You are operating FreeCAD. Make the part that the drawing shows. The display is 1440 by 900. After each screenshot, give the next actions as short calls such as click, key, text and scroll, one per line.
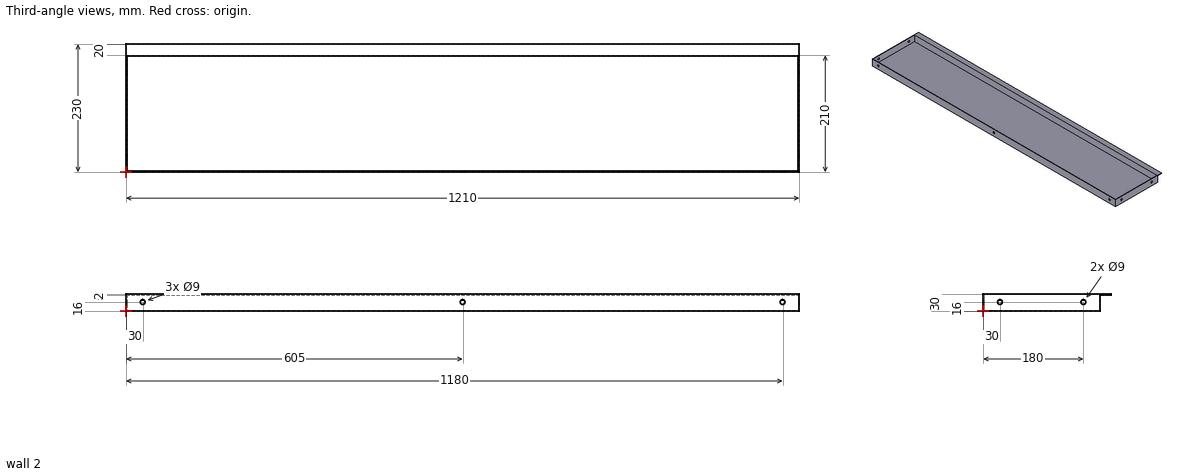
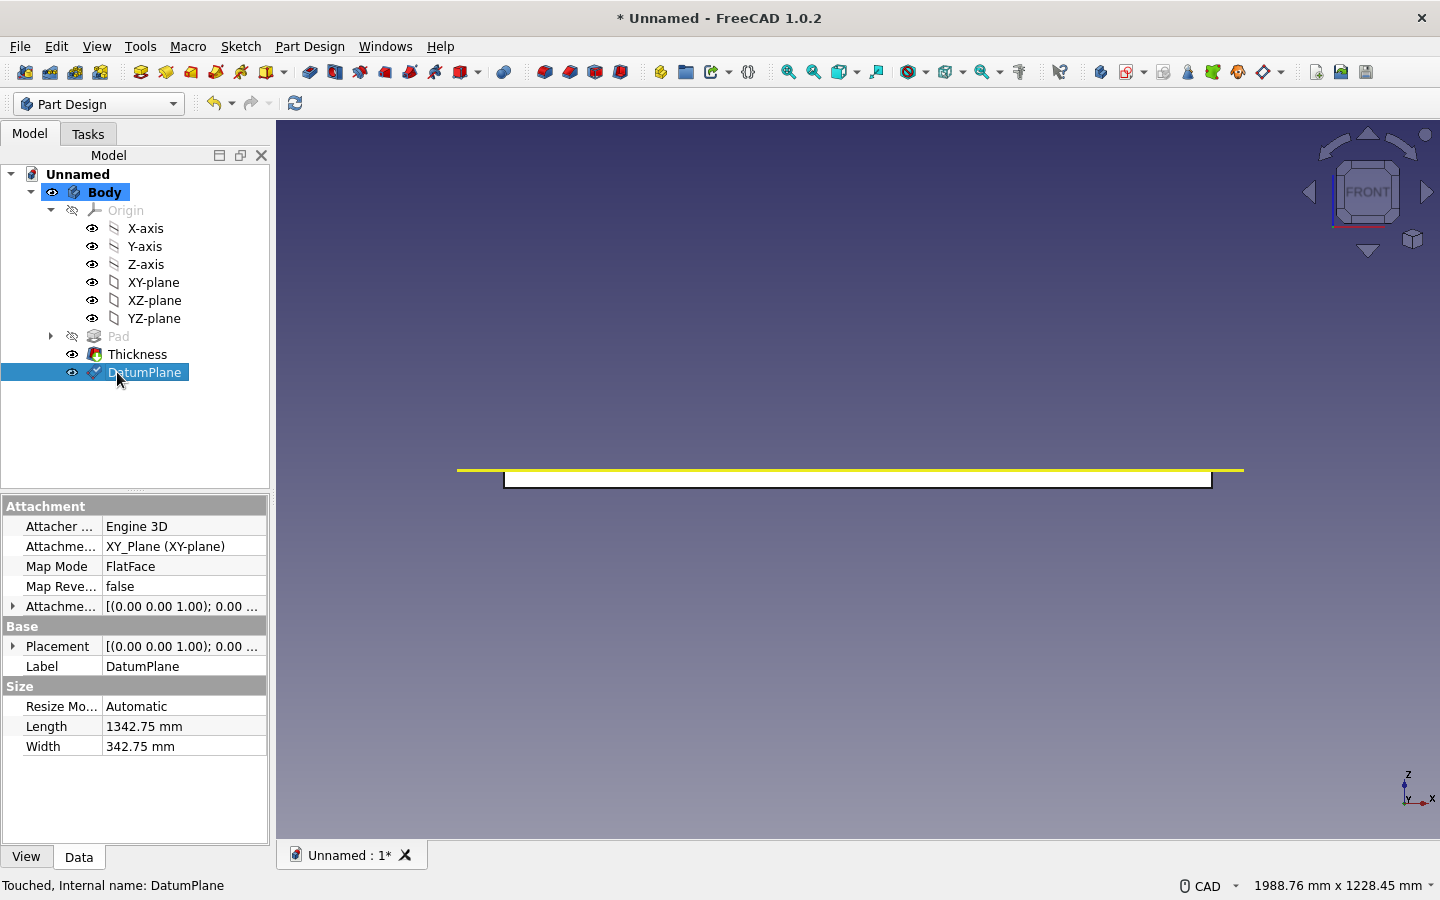
click(1126, 72)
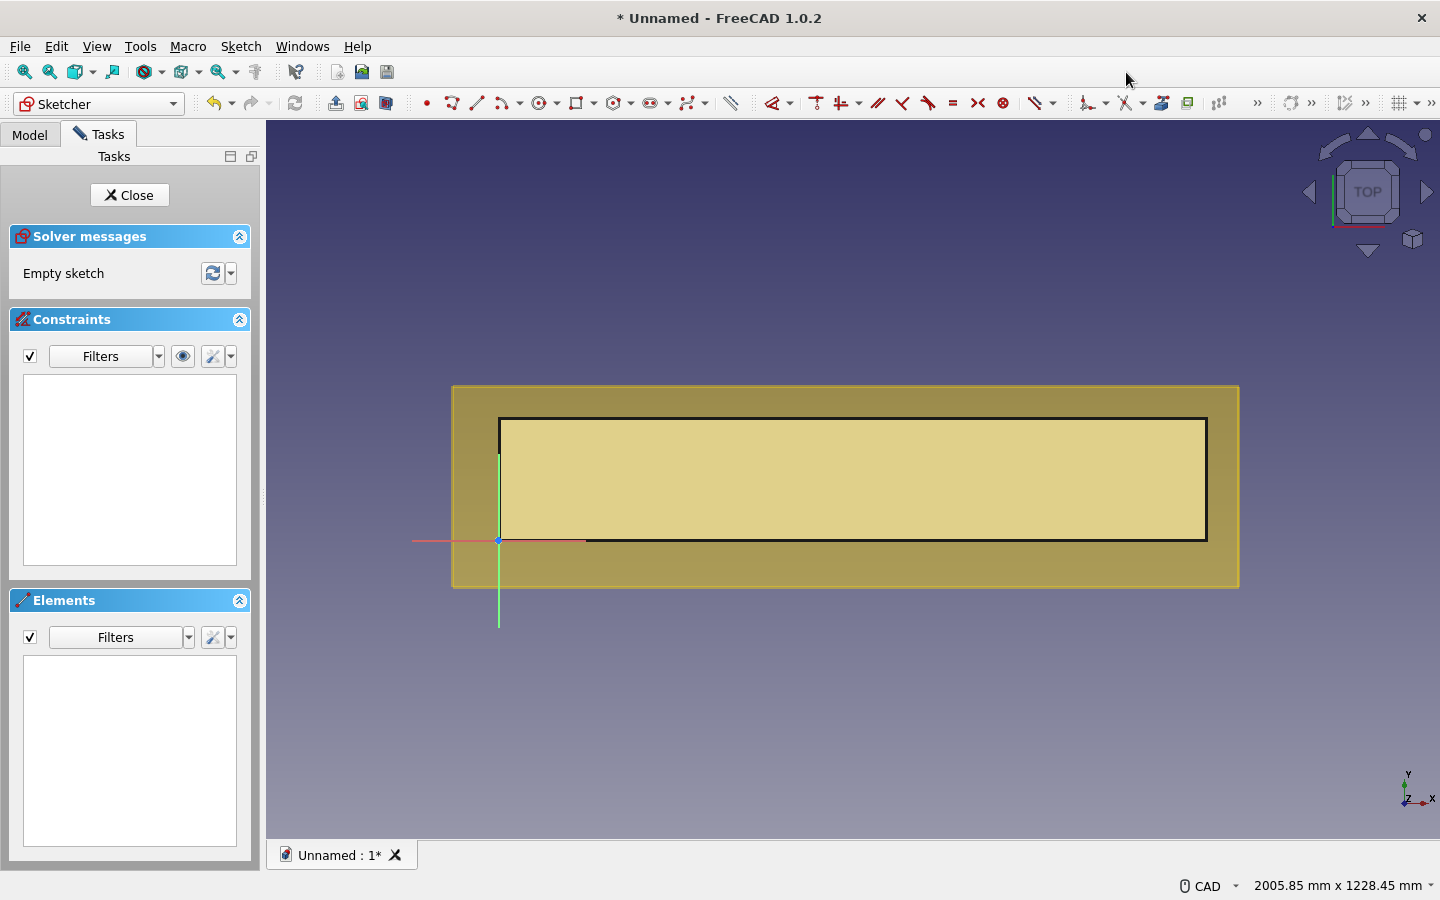
click(576, 104)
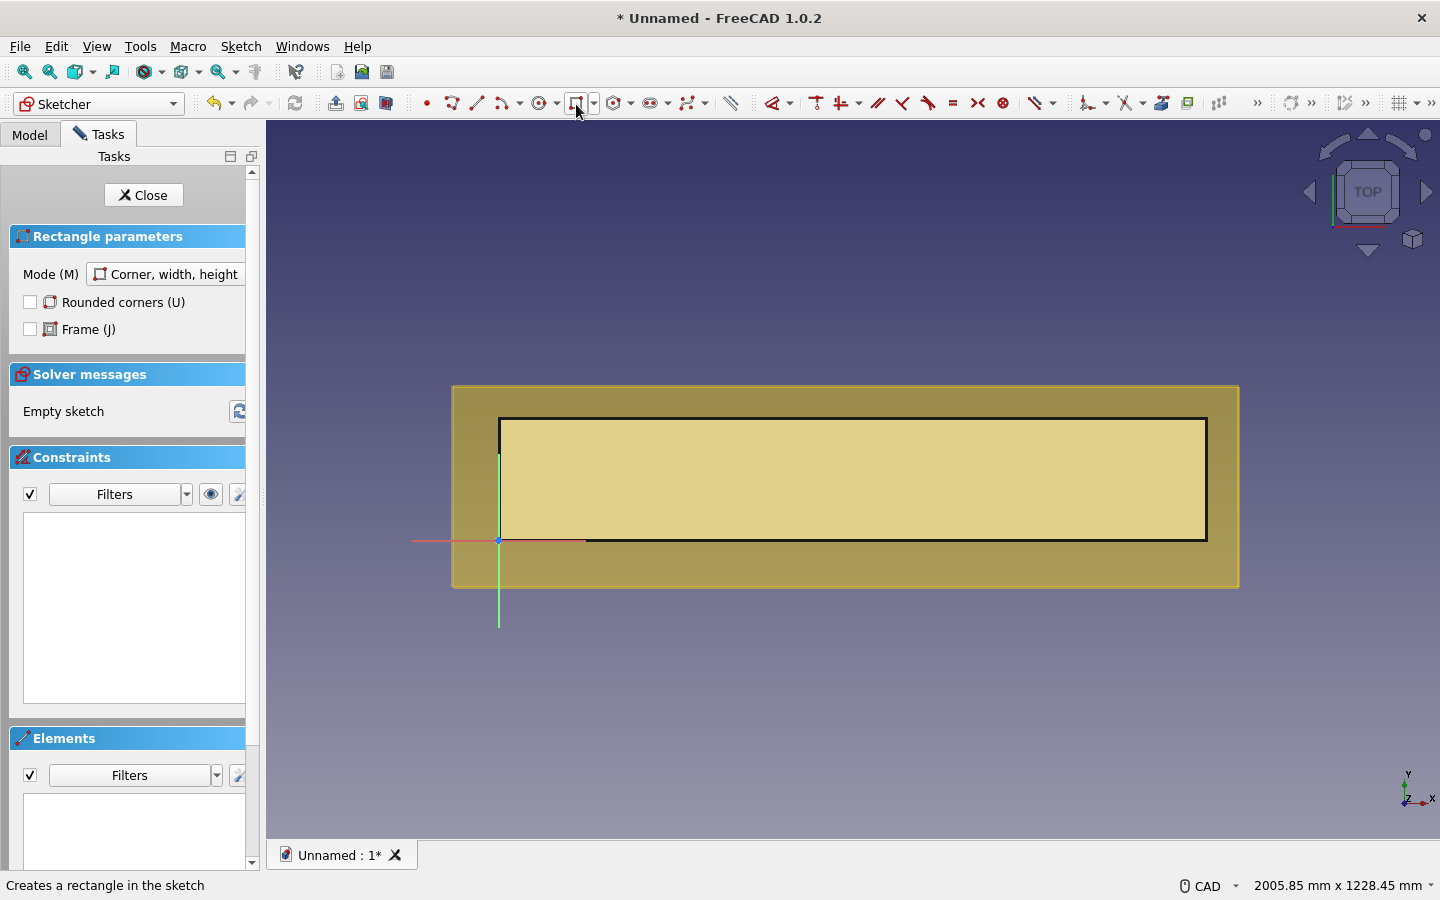
scroll(499, 406, up, 2)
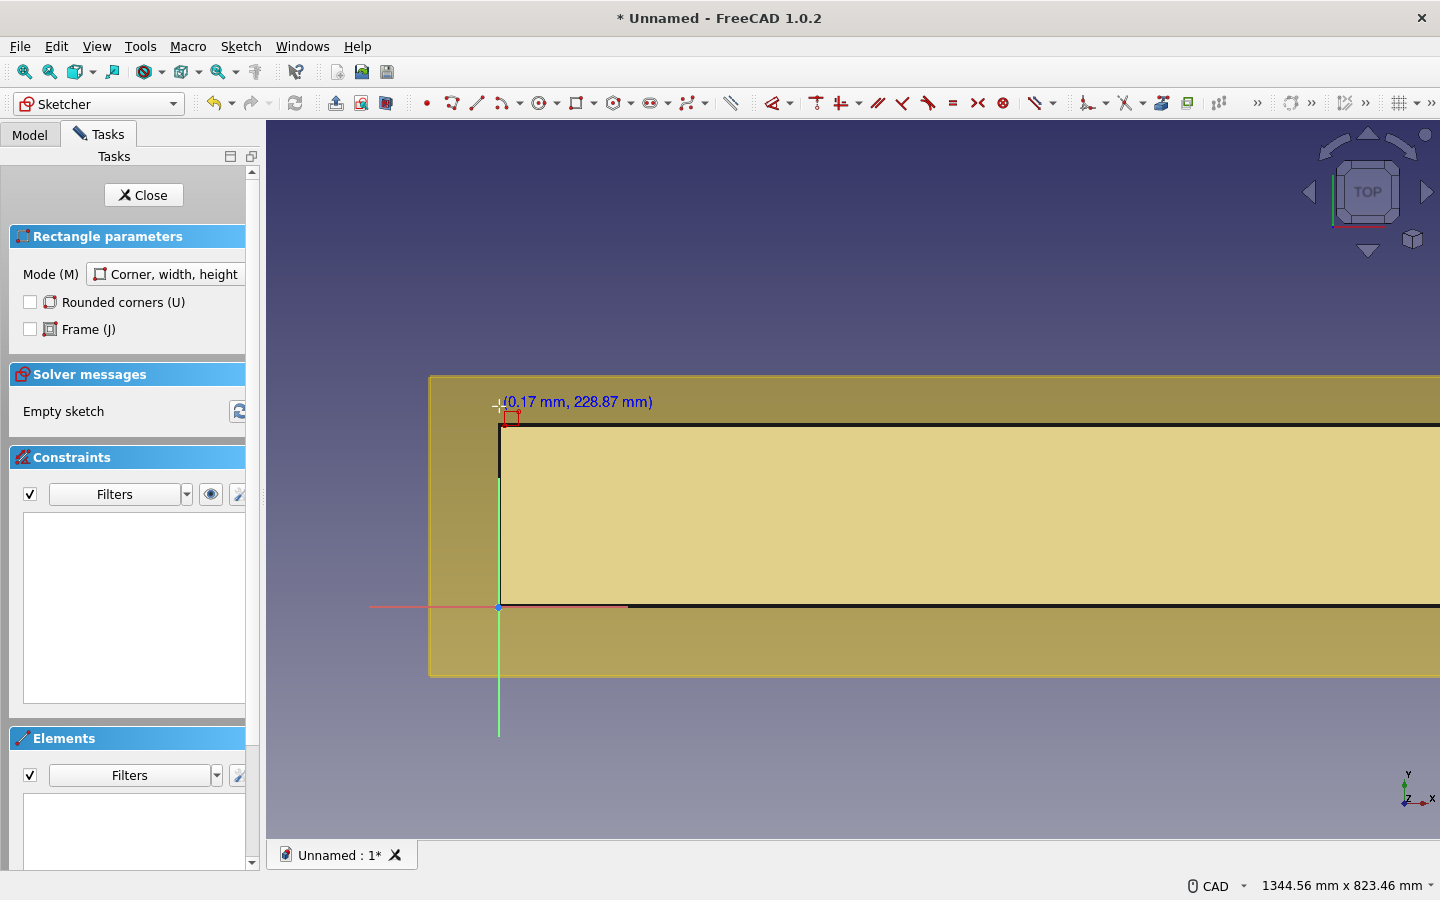
click(499, 406)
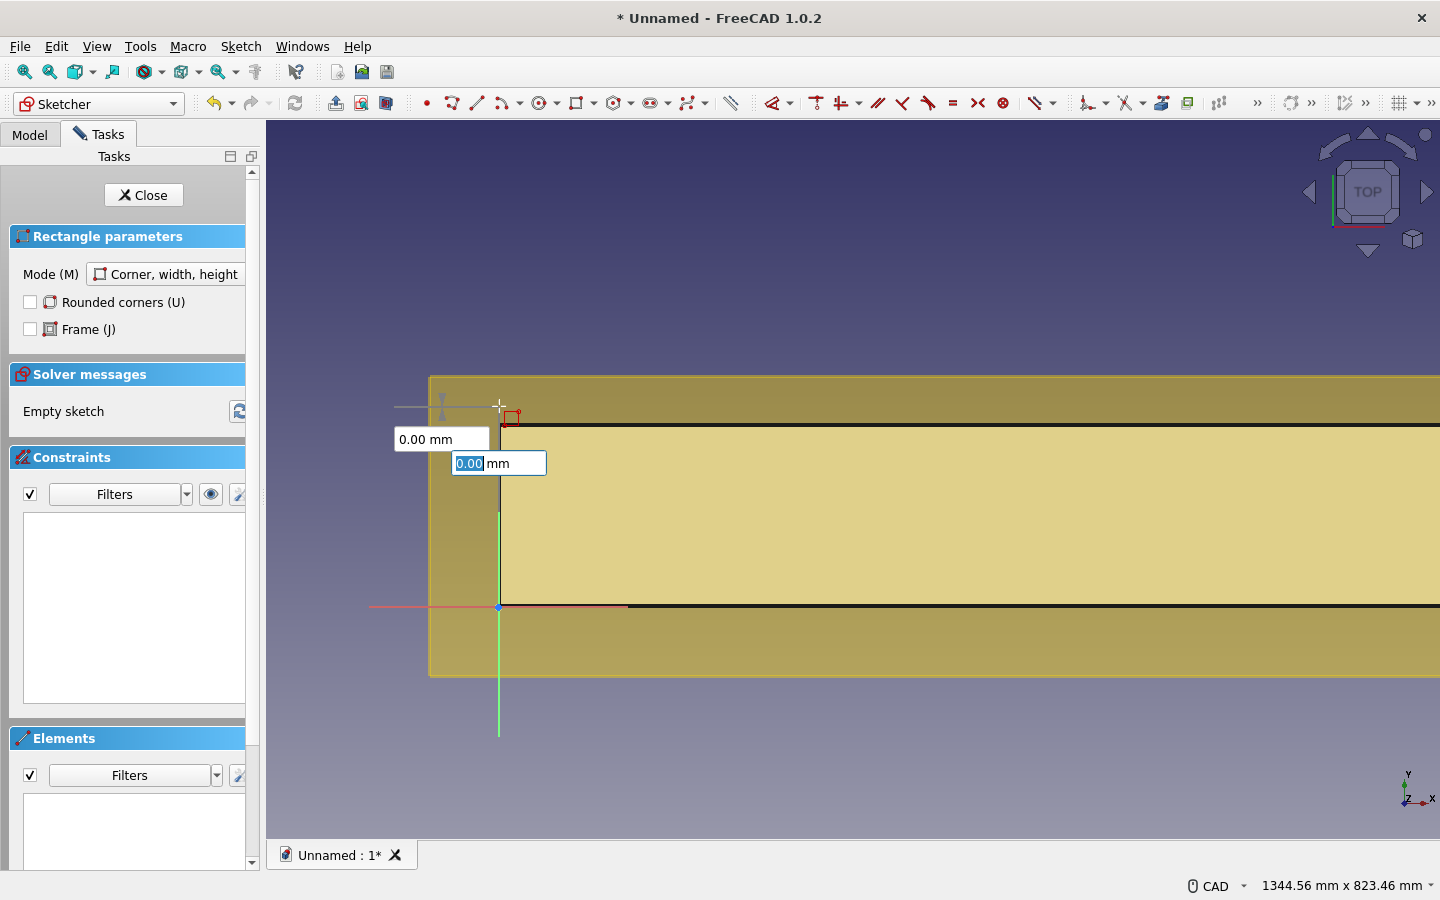
scroll(294, 424, down, 2)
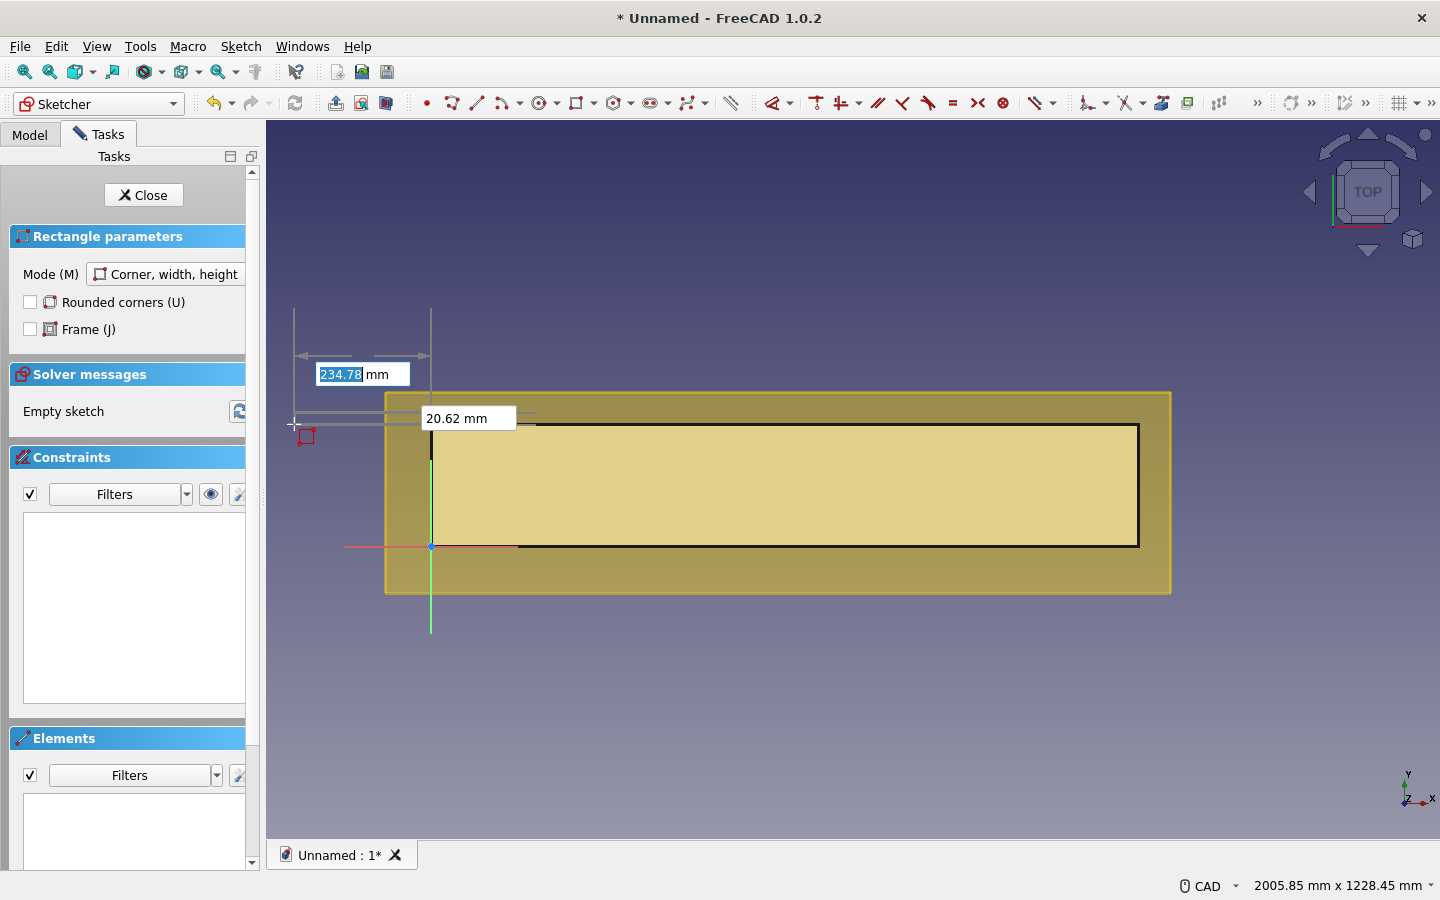
click(1139, 424)
key(Escape)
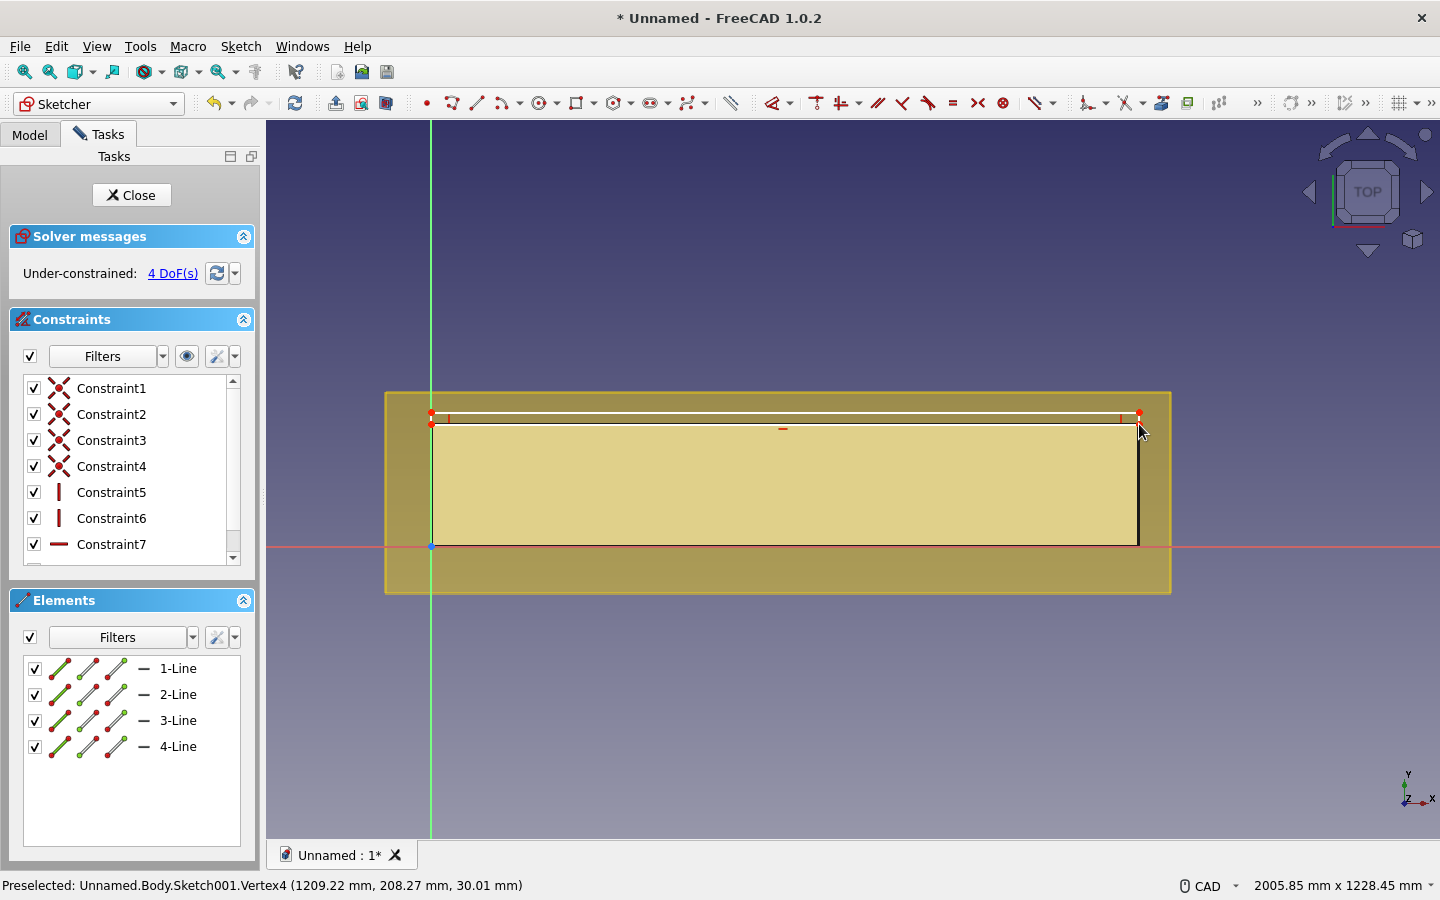
click(431, 413)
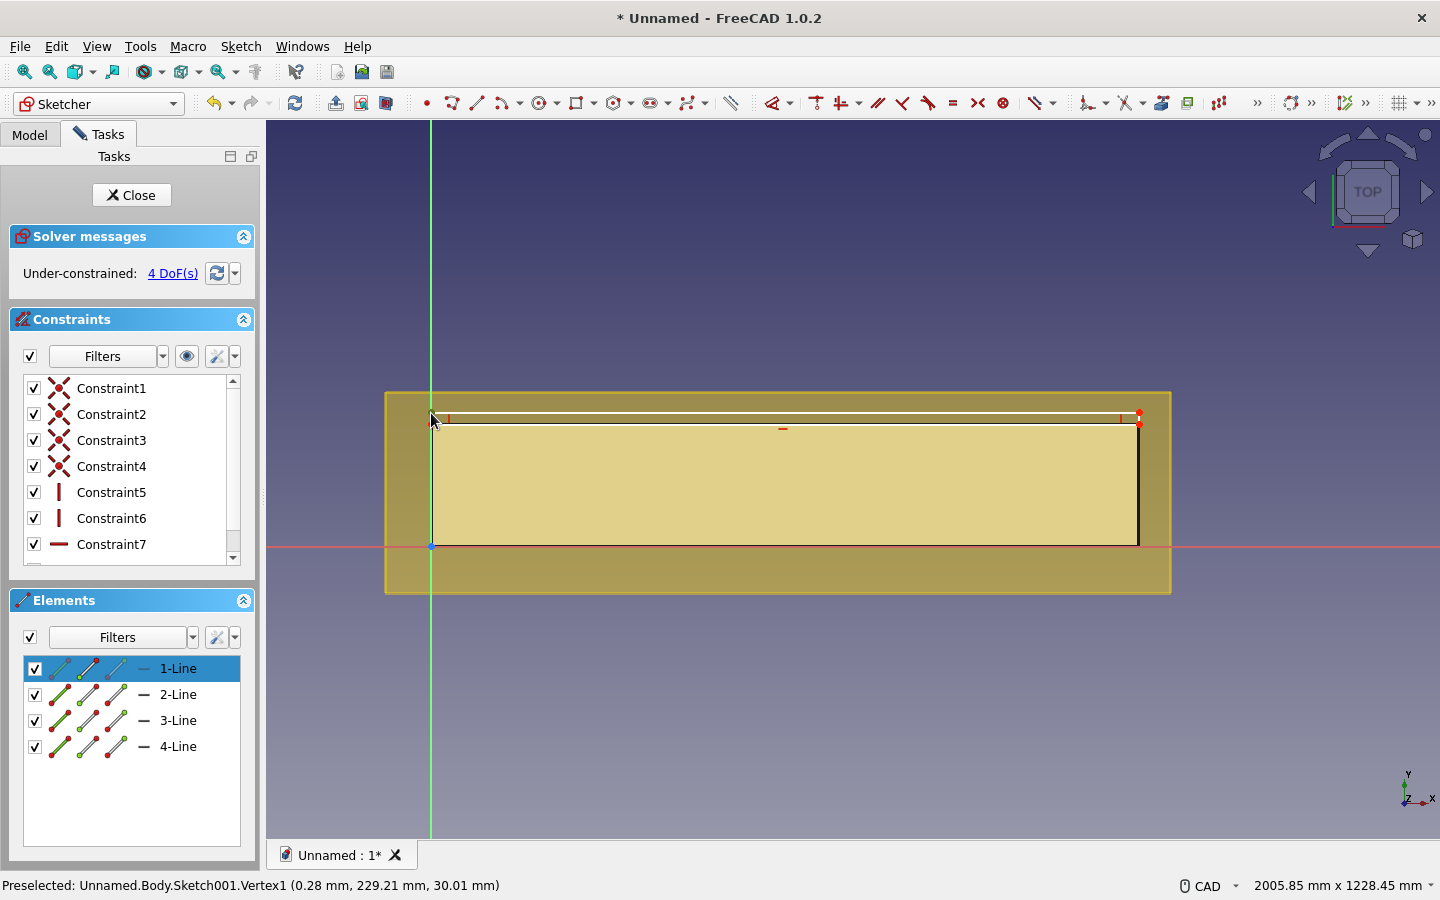
click(431, 764)